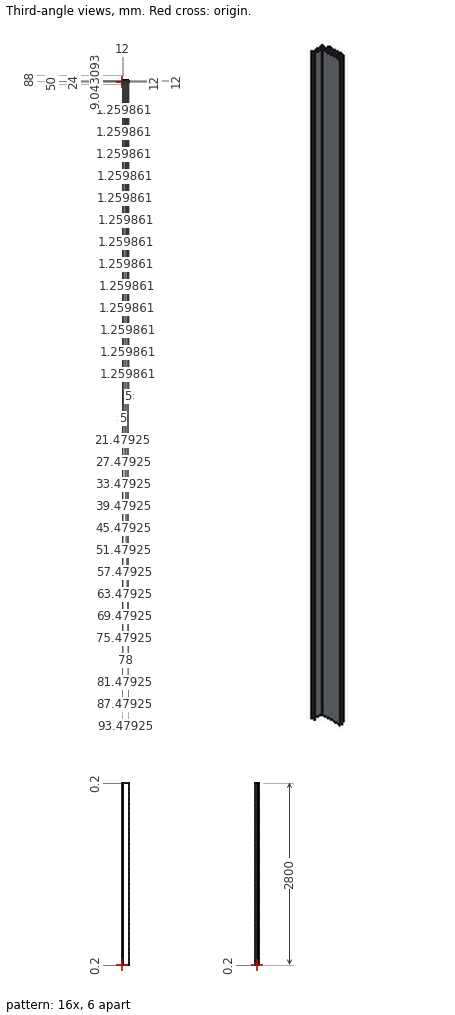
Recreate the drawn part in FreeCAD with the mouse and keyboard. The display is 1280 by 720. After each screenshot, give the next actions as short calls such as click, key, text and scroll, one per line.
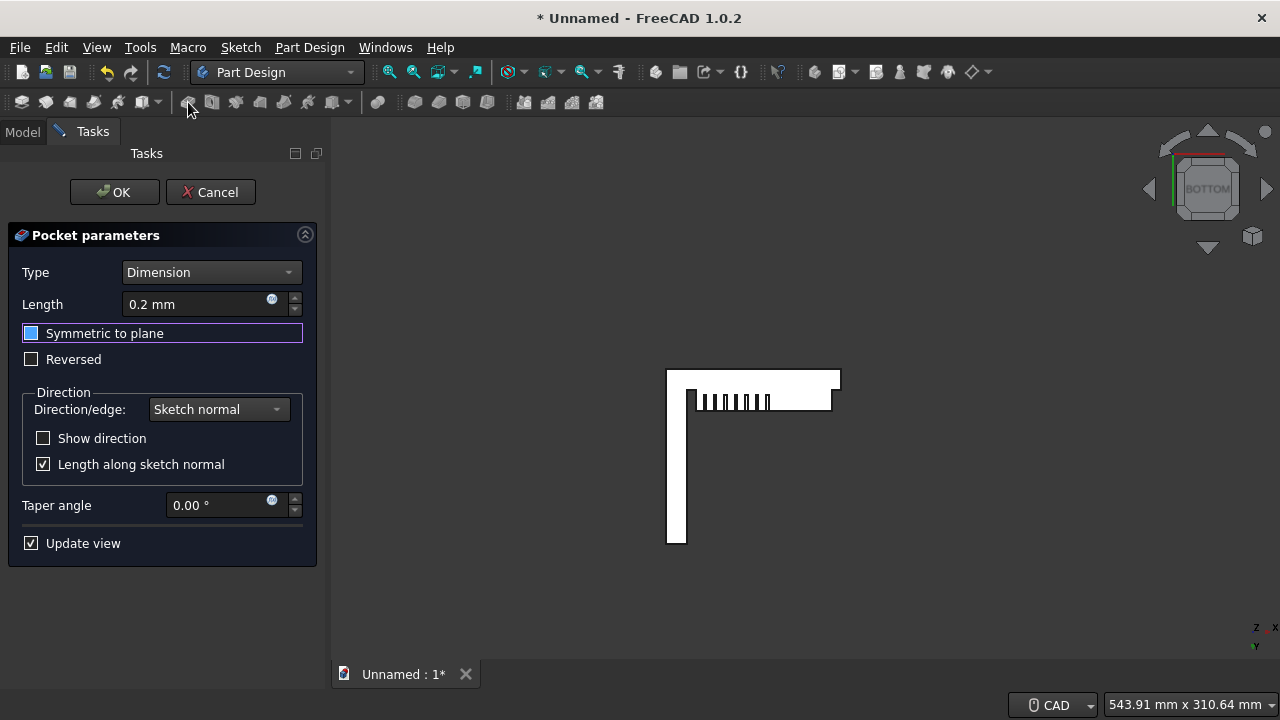
click(115, 192)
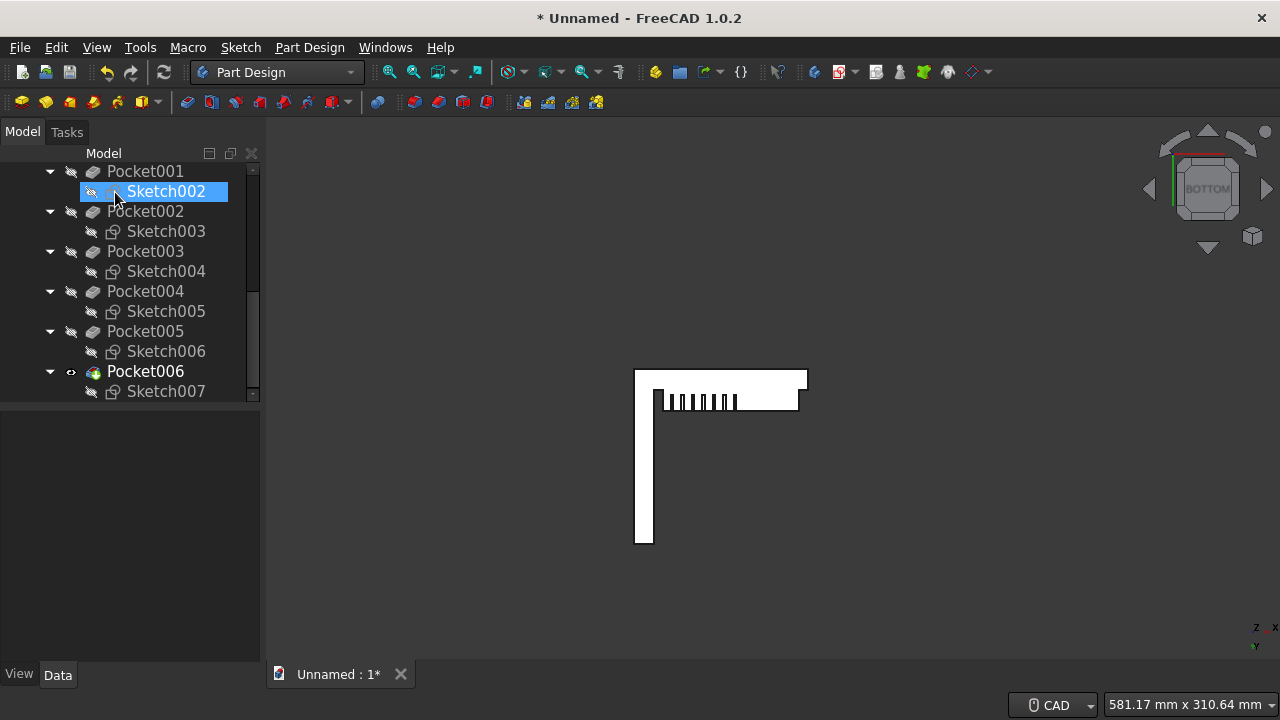
click(390, 72)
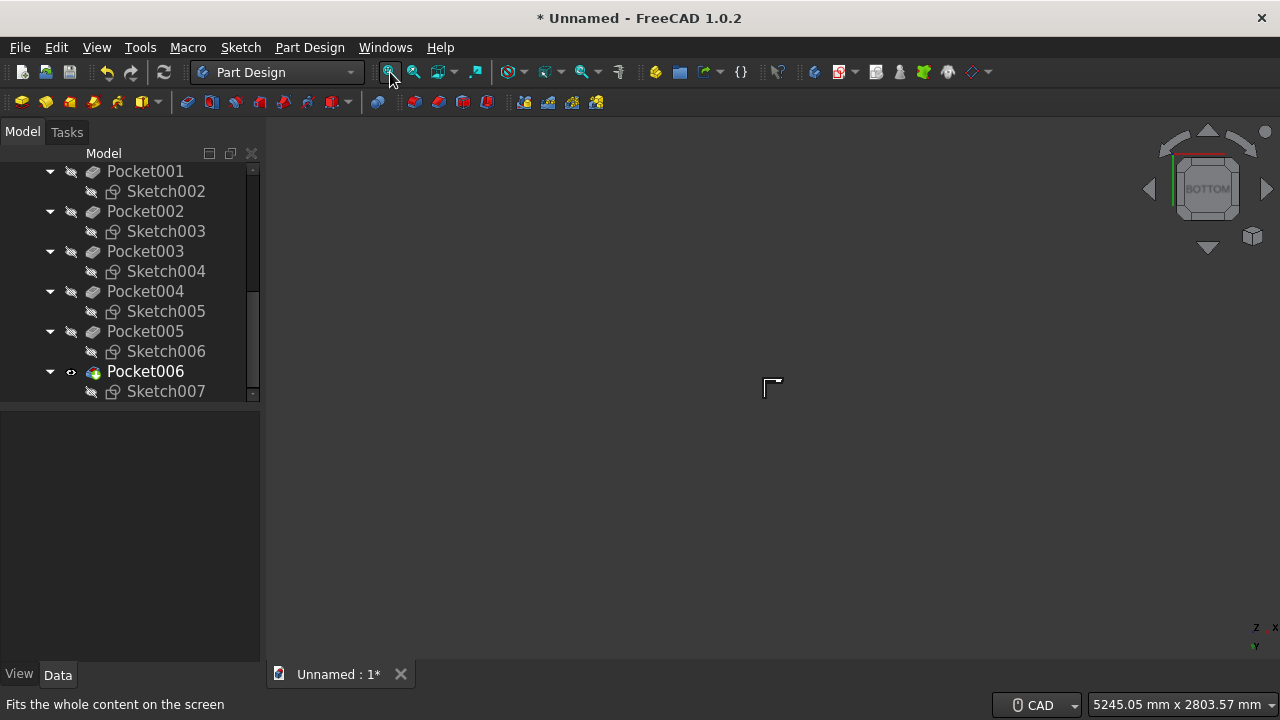
click(840, 72)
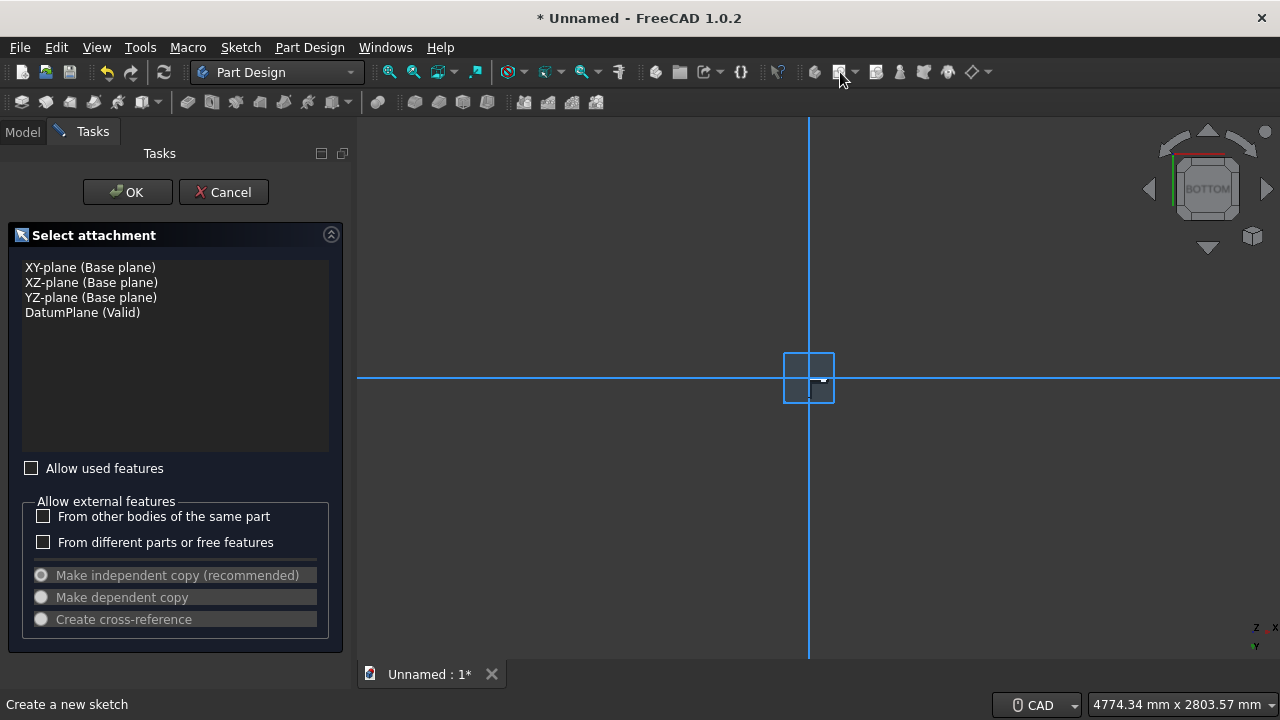
click(82, 268)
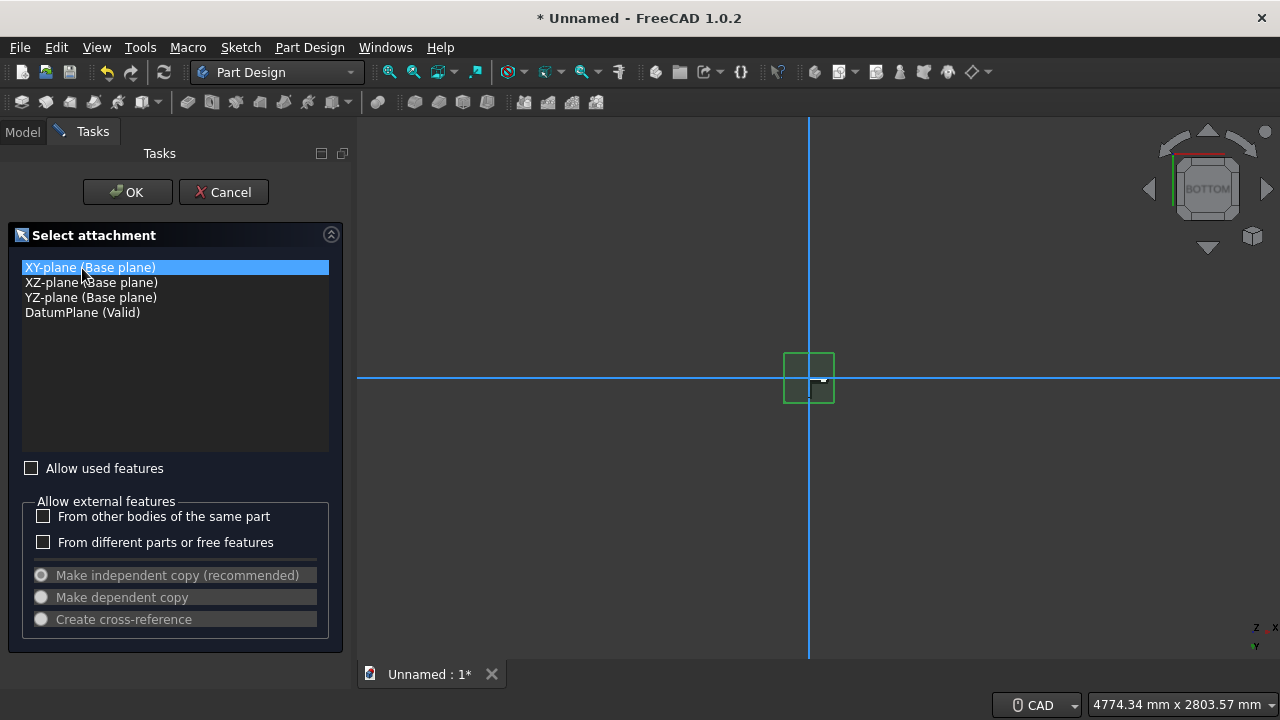
click(128, 192)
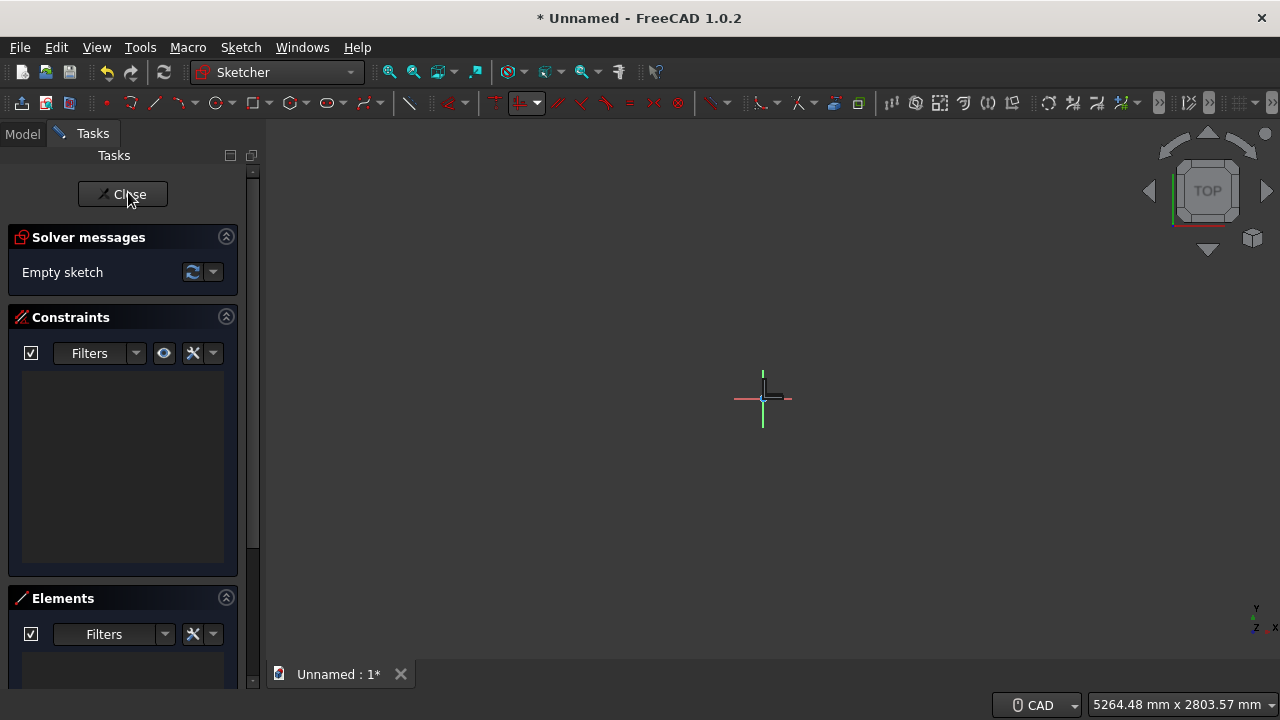
click(70, 104)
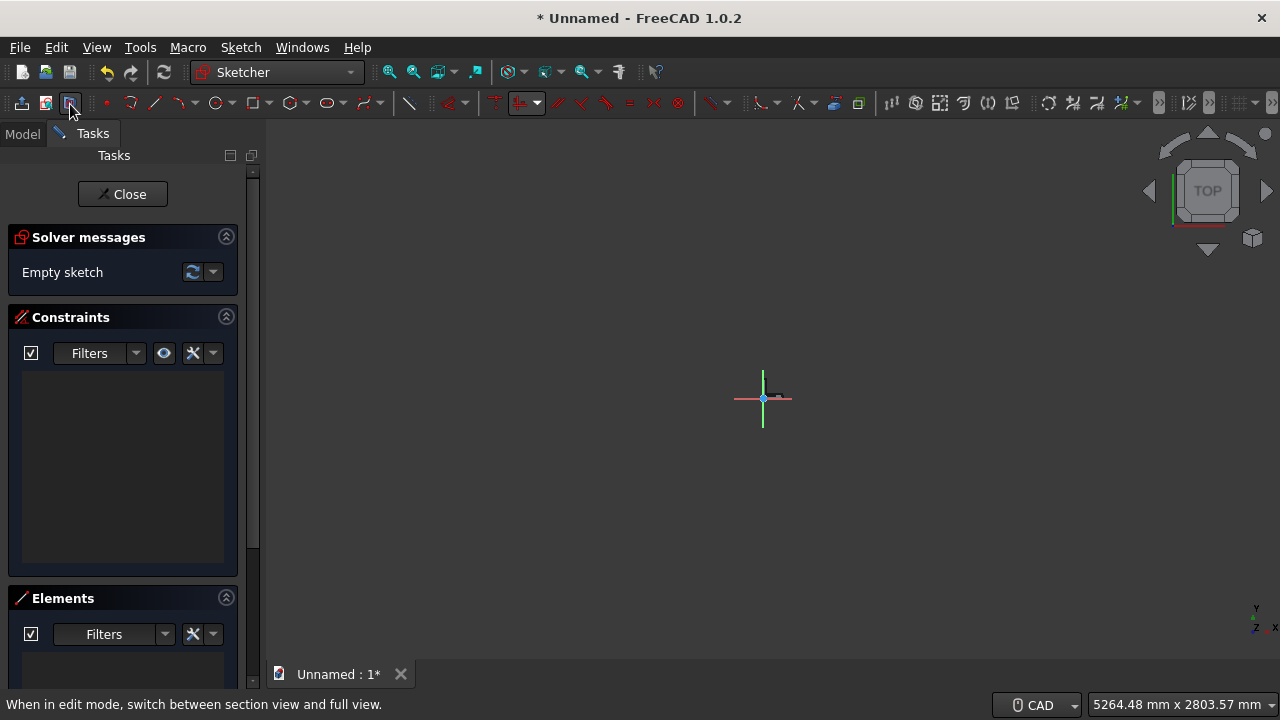
scroll(779, 395, up, 15)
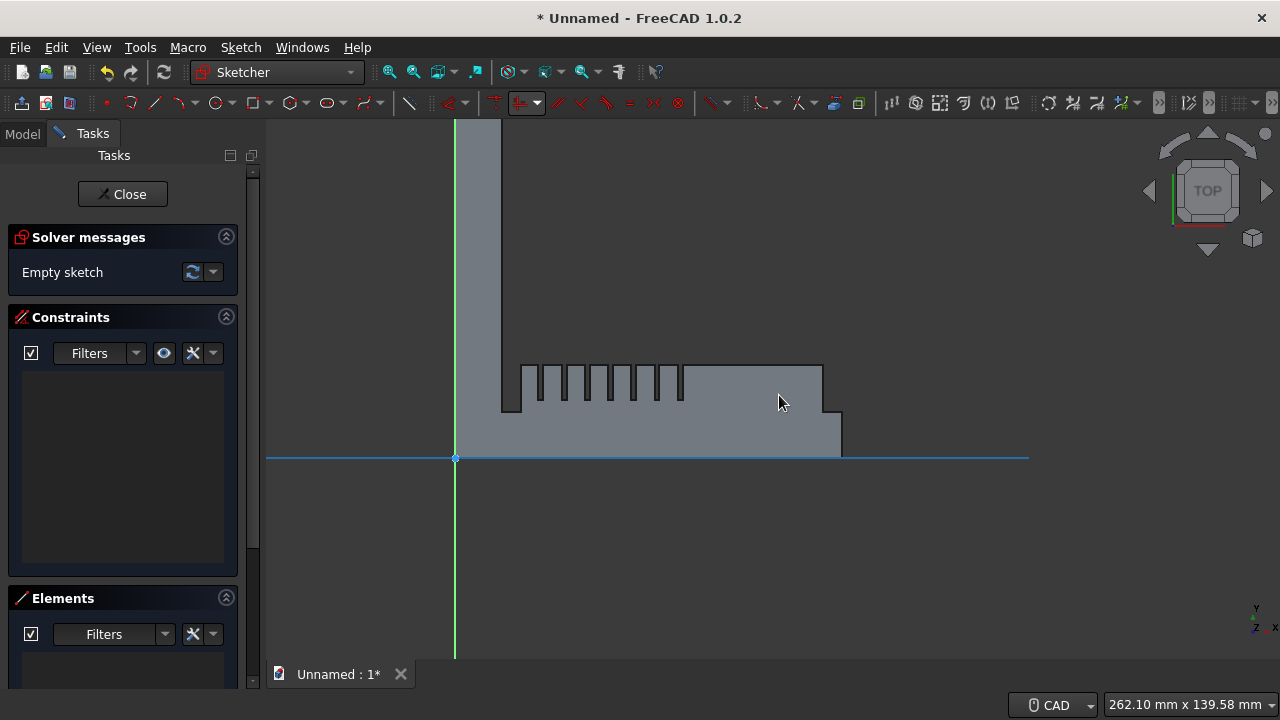
scroll(703, 382, up, 11)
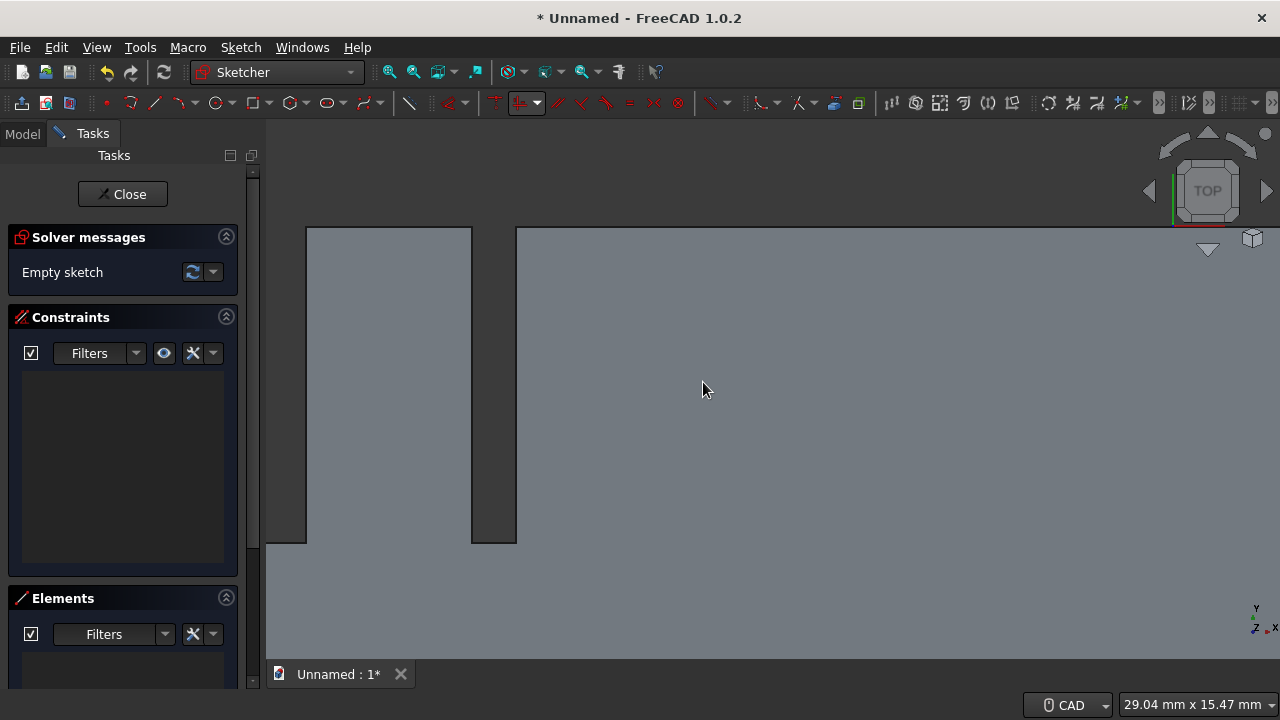
click(254, 104)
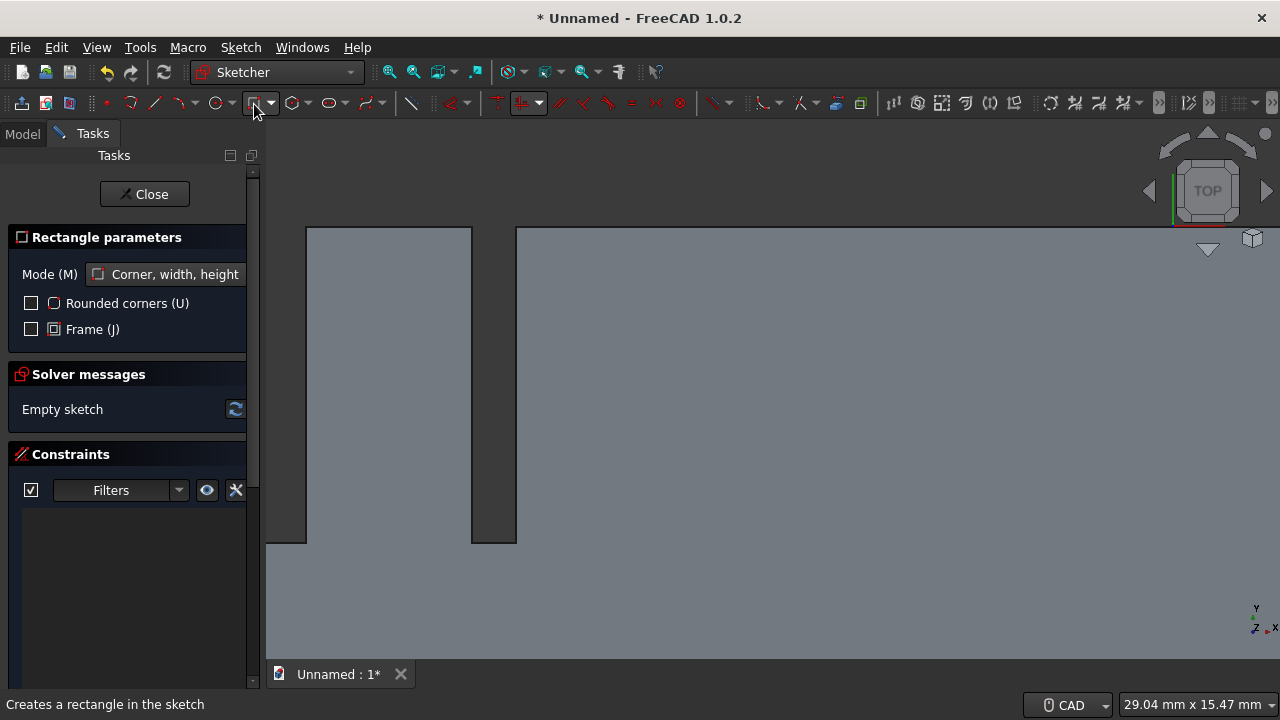
click(681, 227)
move(725, 543)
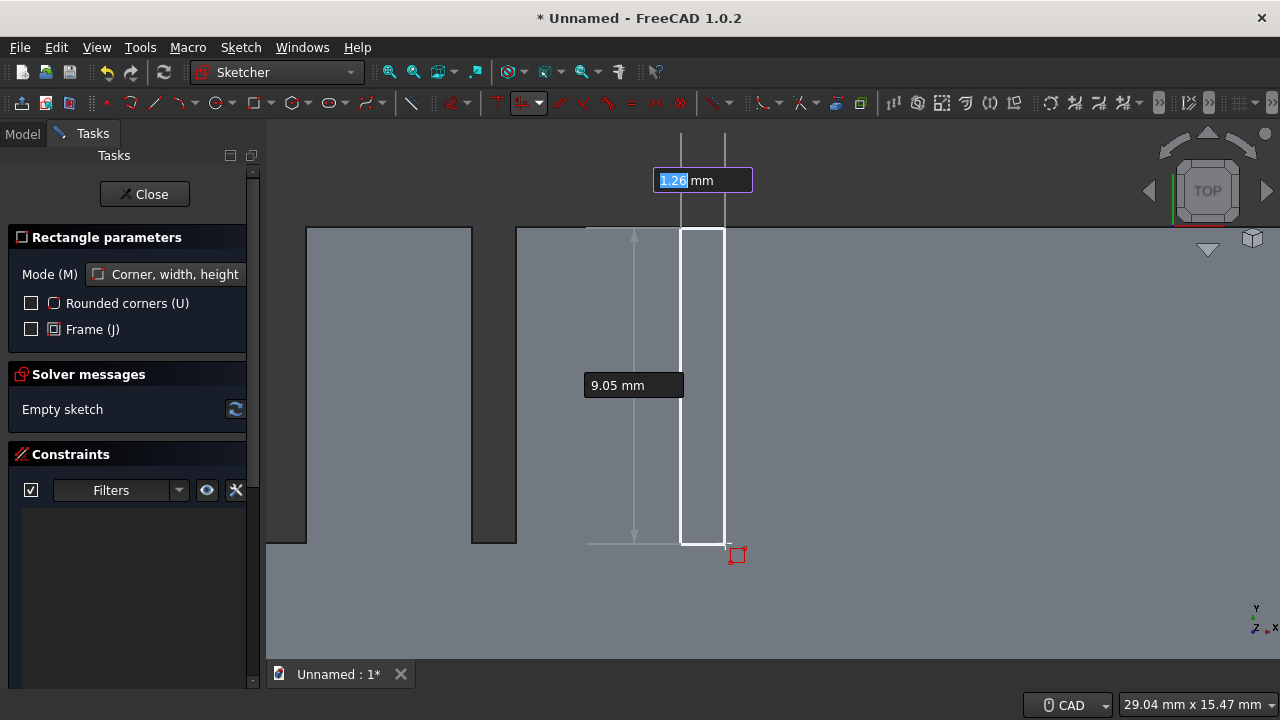
text(1.259861)
key(Tab)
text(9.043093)
key(Return)
key(Escape)